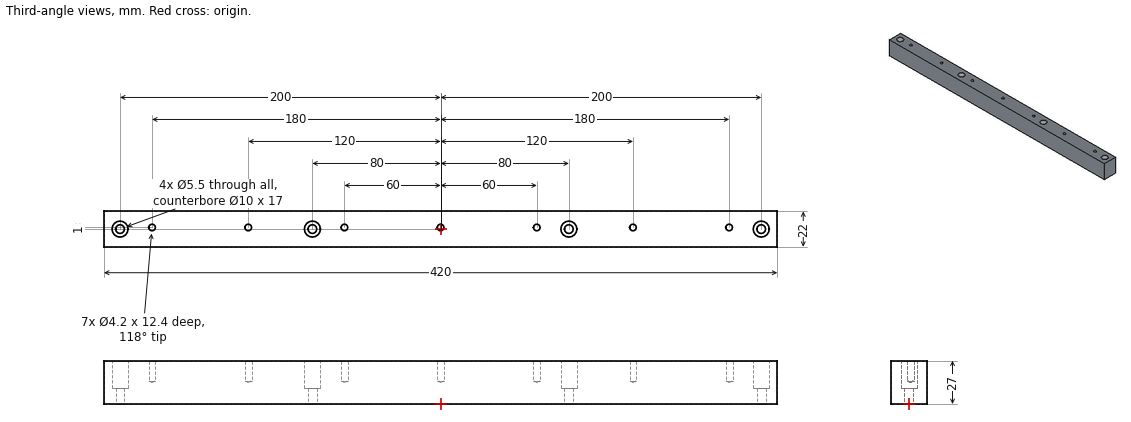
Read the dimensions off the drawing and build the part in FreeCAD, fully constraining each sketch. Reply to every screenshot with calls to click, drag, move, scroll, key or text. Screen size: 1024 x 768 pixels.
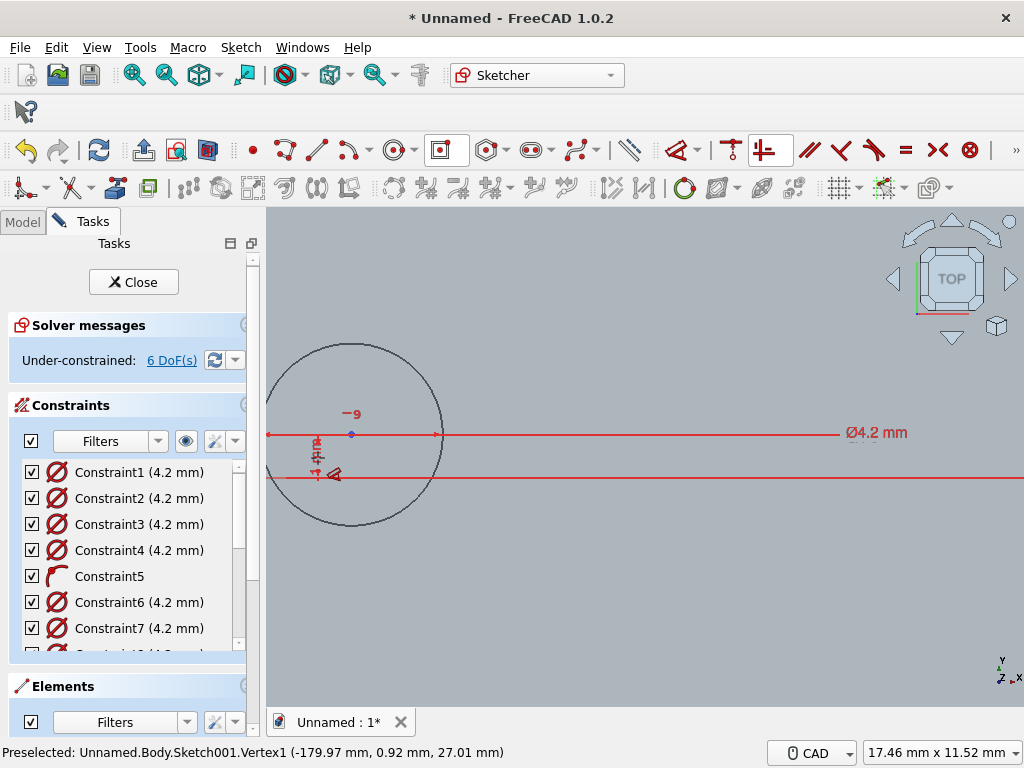
scroll(363, 458, down, 18)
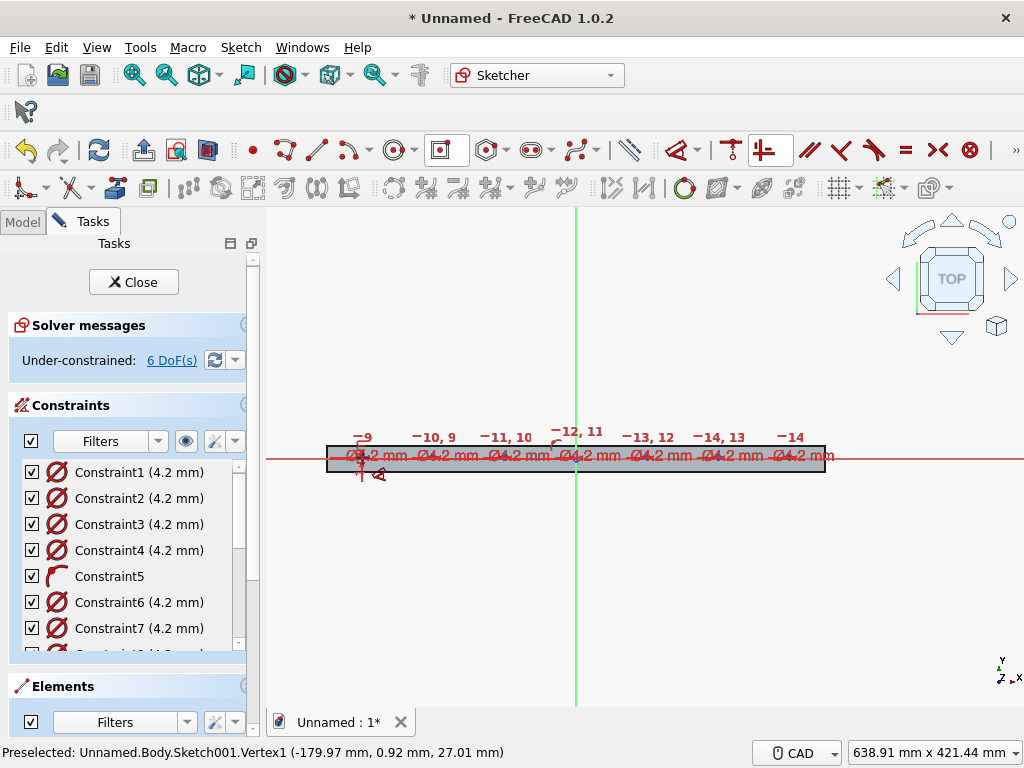
click(505, 458)
click(541, 493)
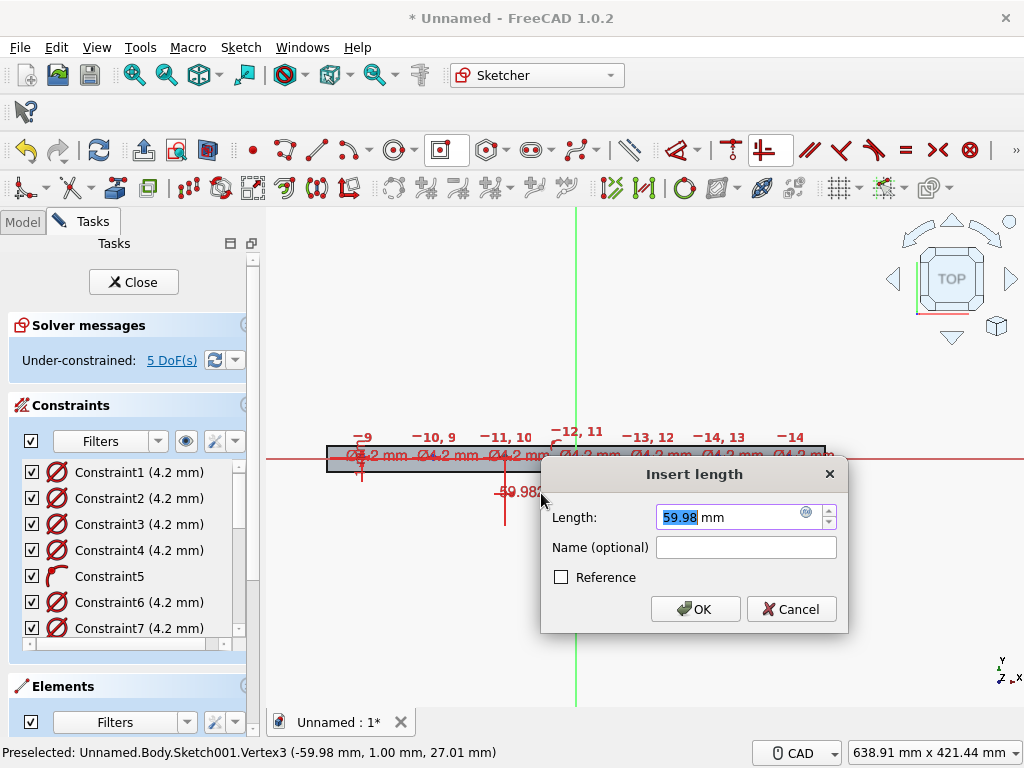
text(60)
key(Return)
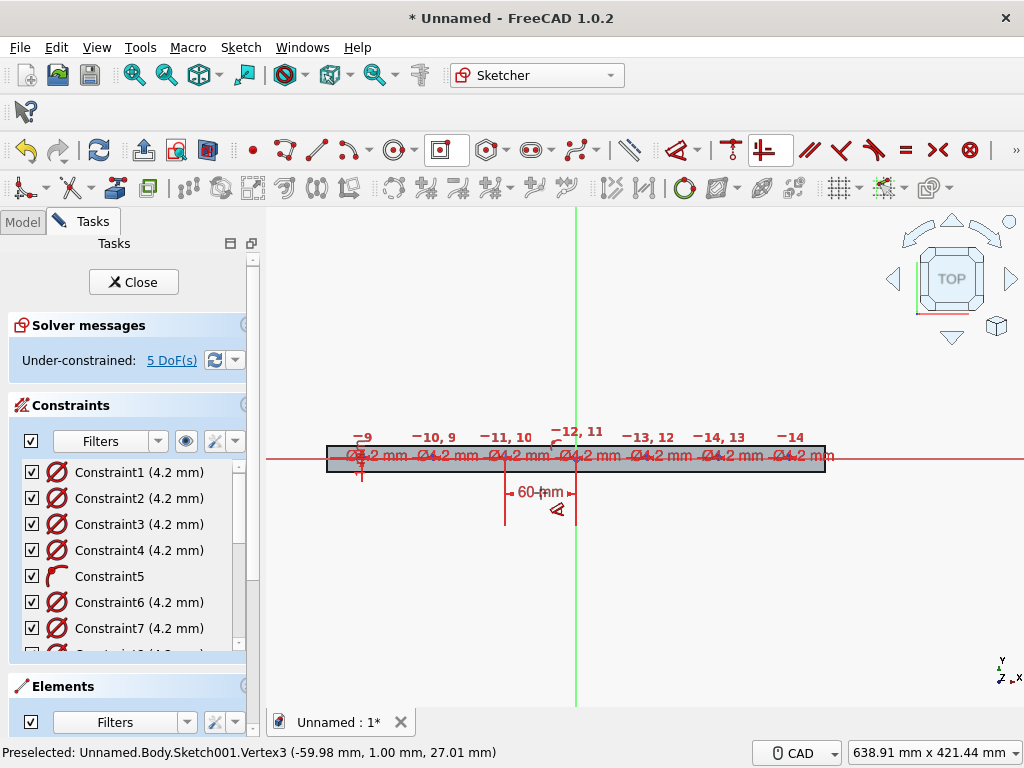
click(647, 458)
click(612, 493)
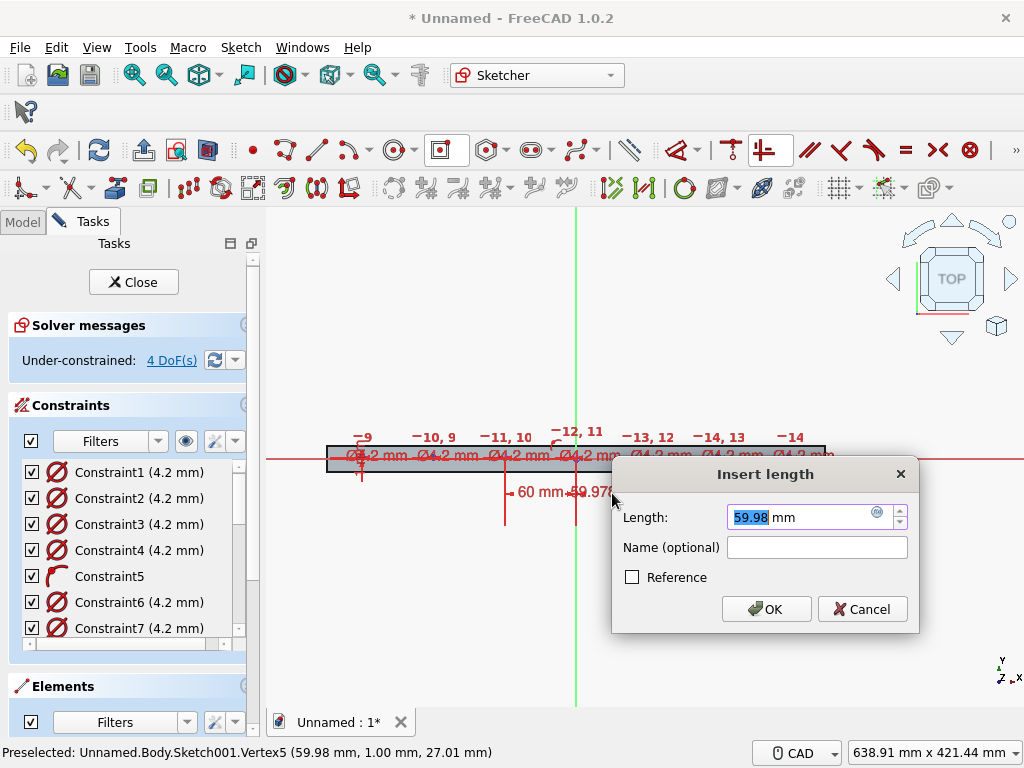
text(60)
key(Return)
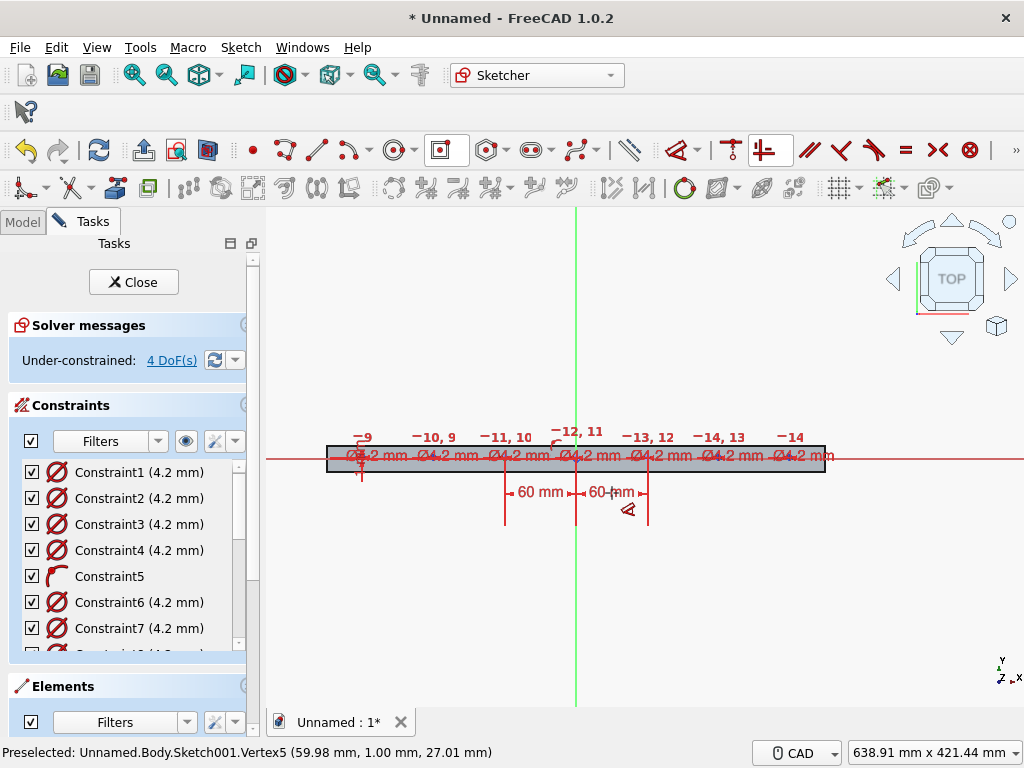
click(363, 458)
click(470, 493)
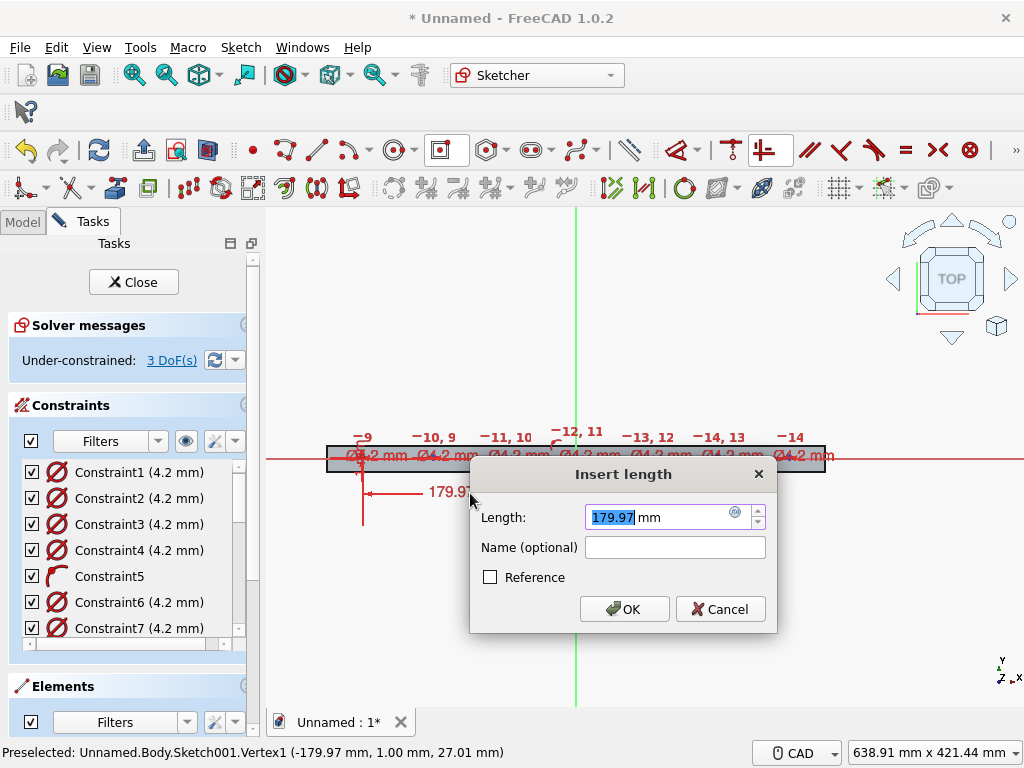
text(180)
key(Return)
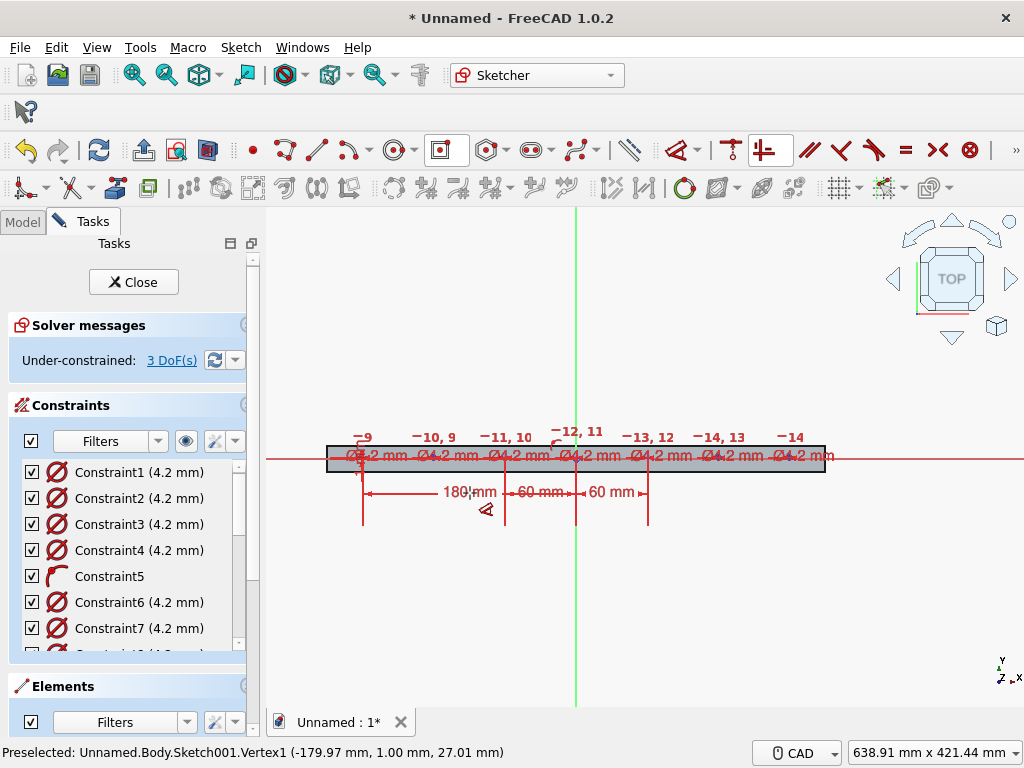
click(434, 458)
click(505, 424)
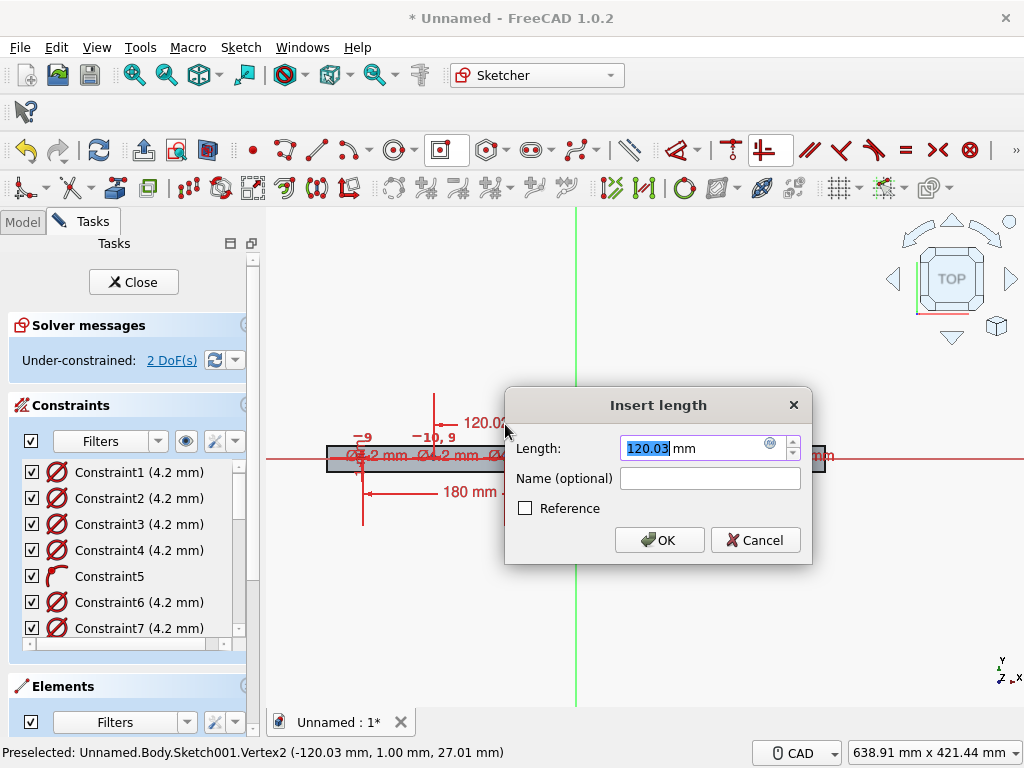
text(120)
key(Return)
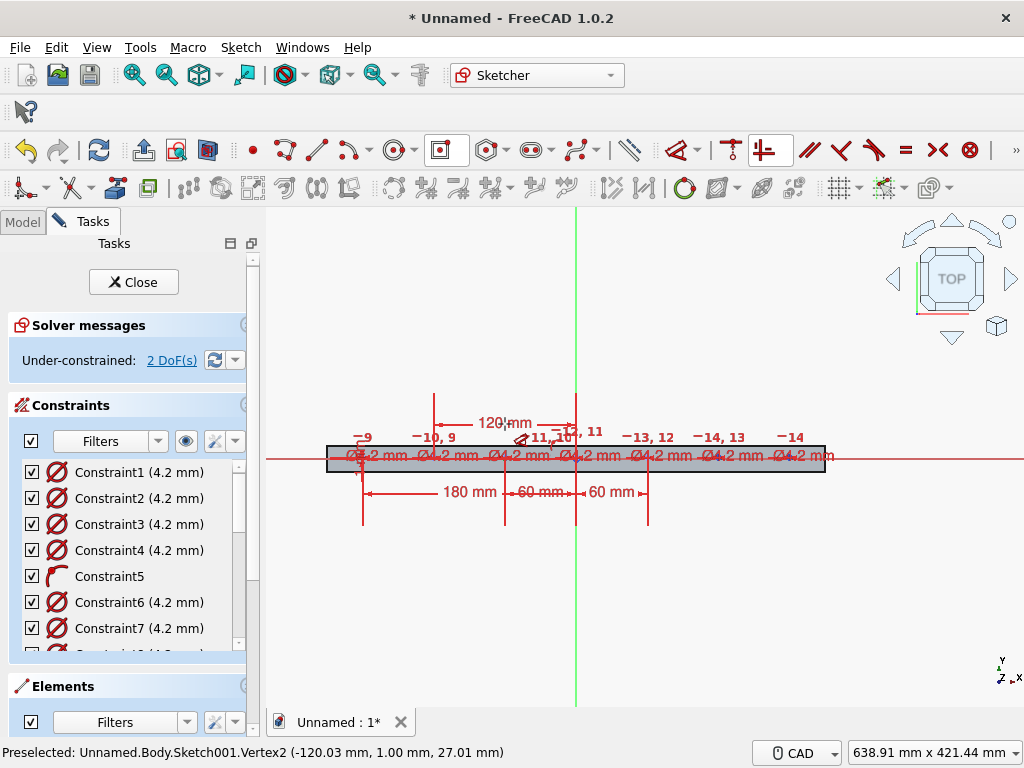
click(719, 458)
click(697, 493)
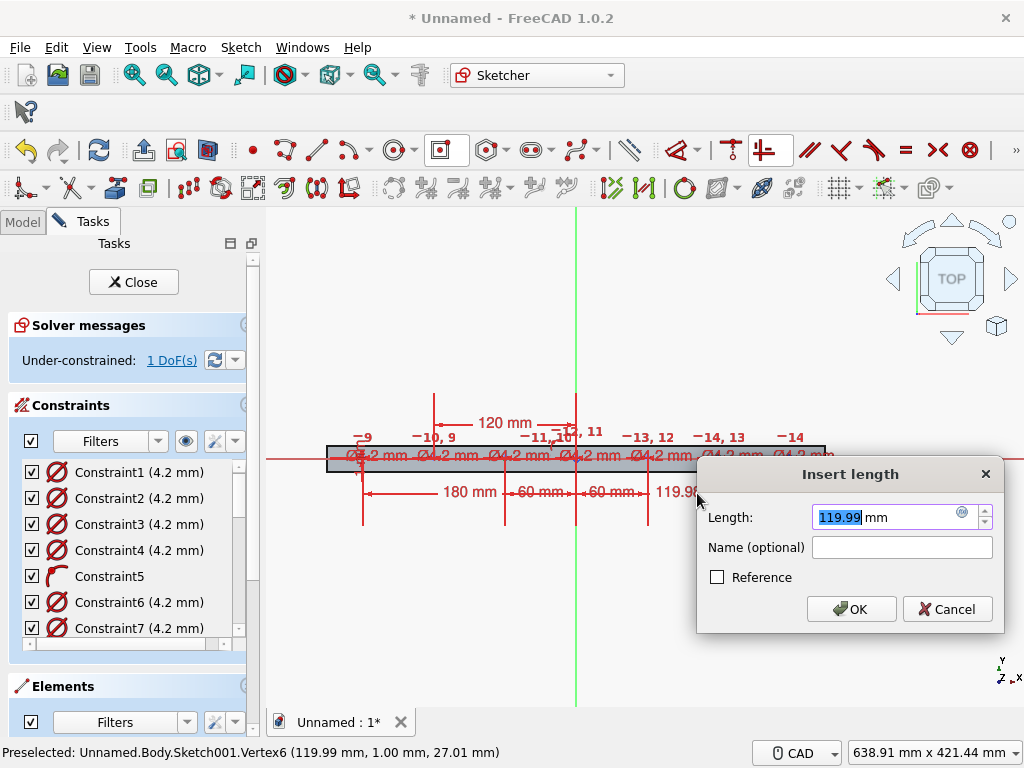
text(120)
key(Return)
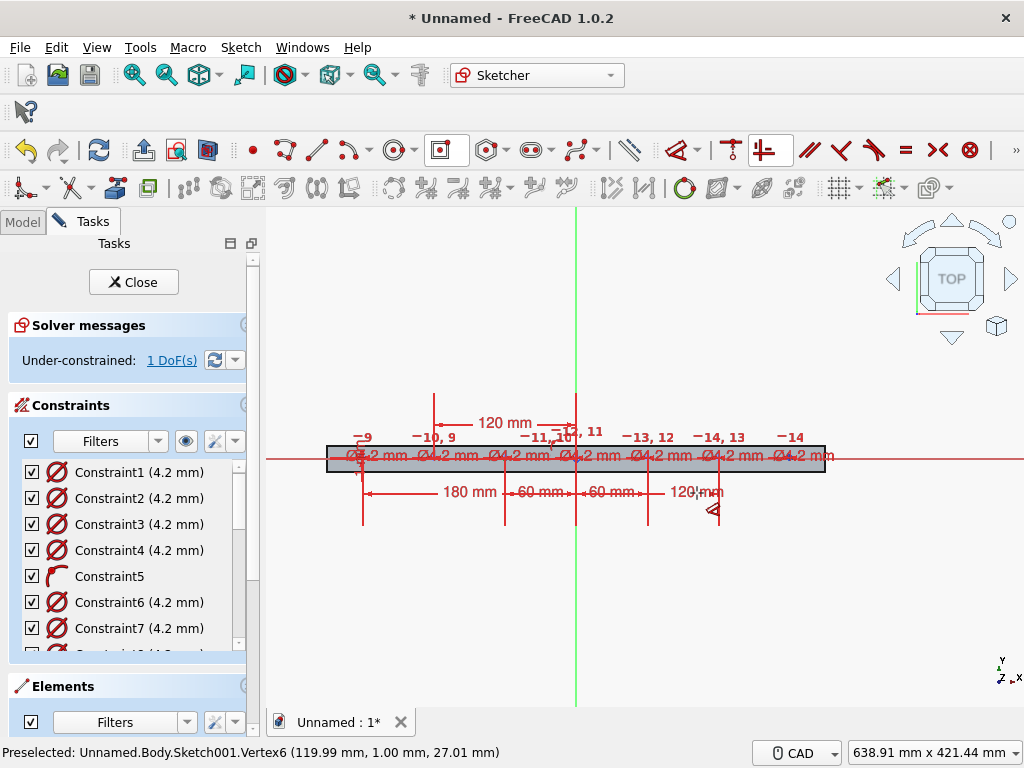
click(790, 458)
click(683, 424)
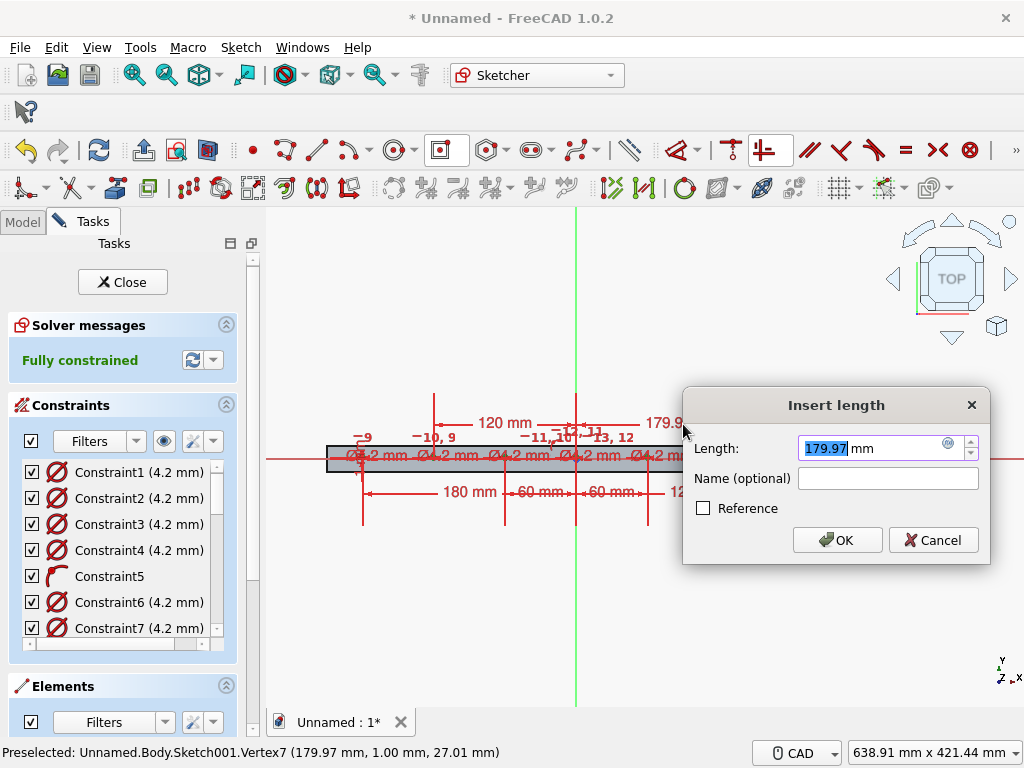
text(180)
key(Return)
key(Escape)